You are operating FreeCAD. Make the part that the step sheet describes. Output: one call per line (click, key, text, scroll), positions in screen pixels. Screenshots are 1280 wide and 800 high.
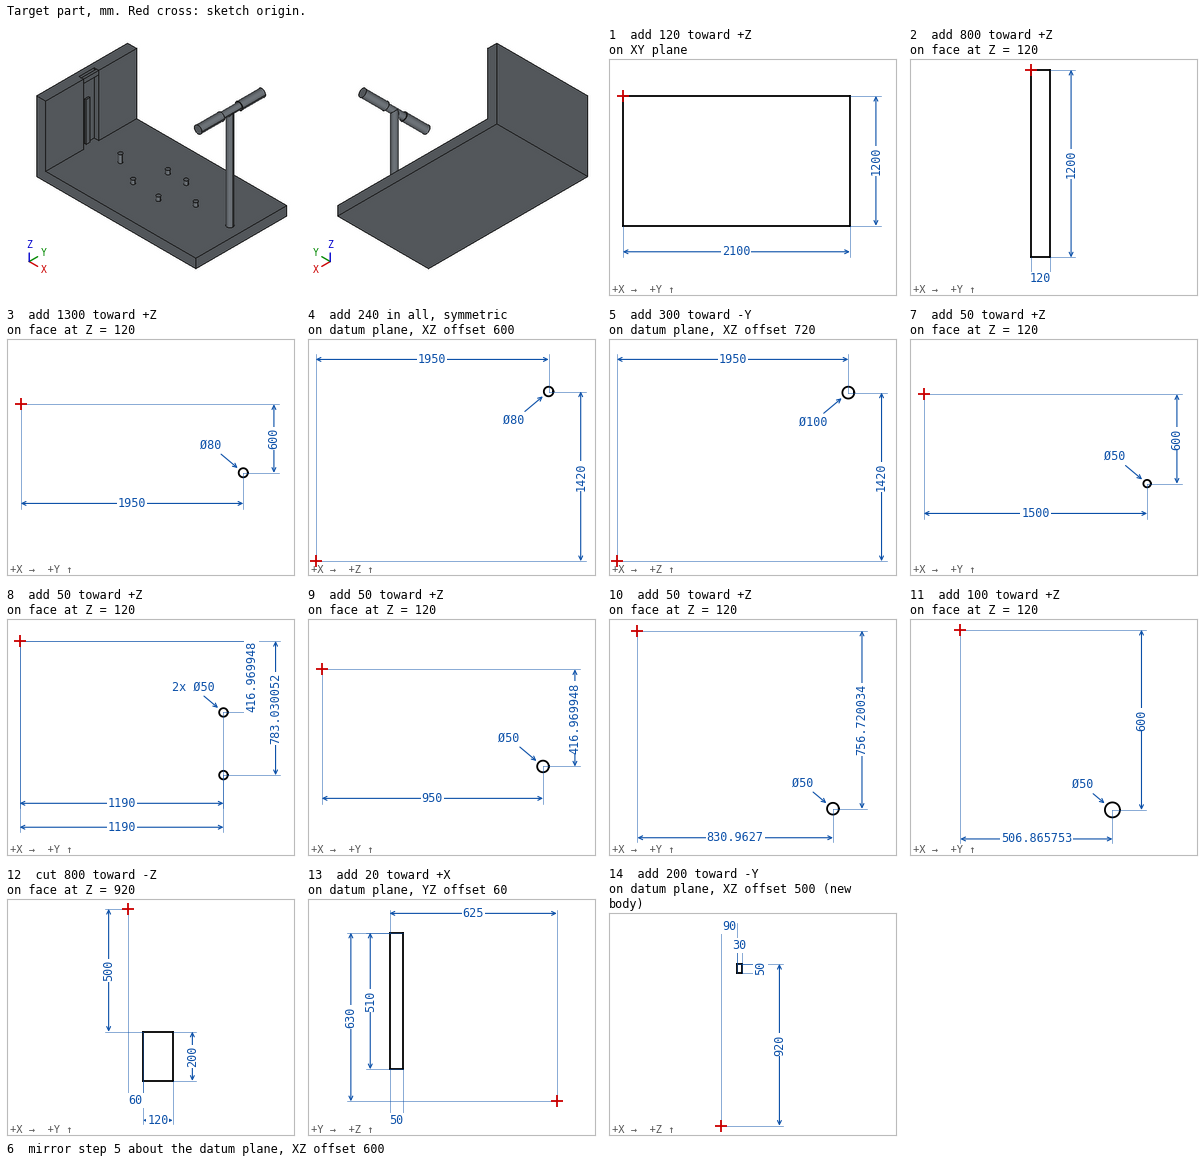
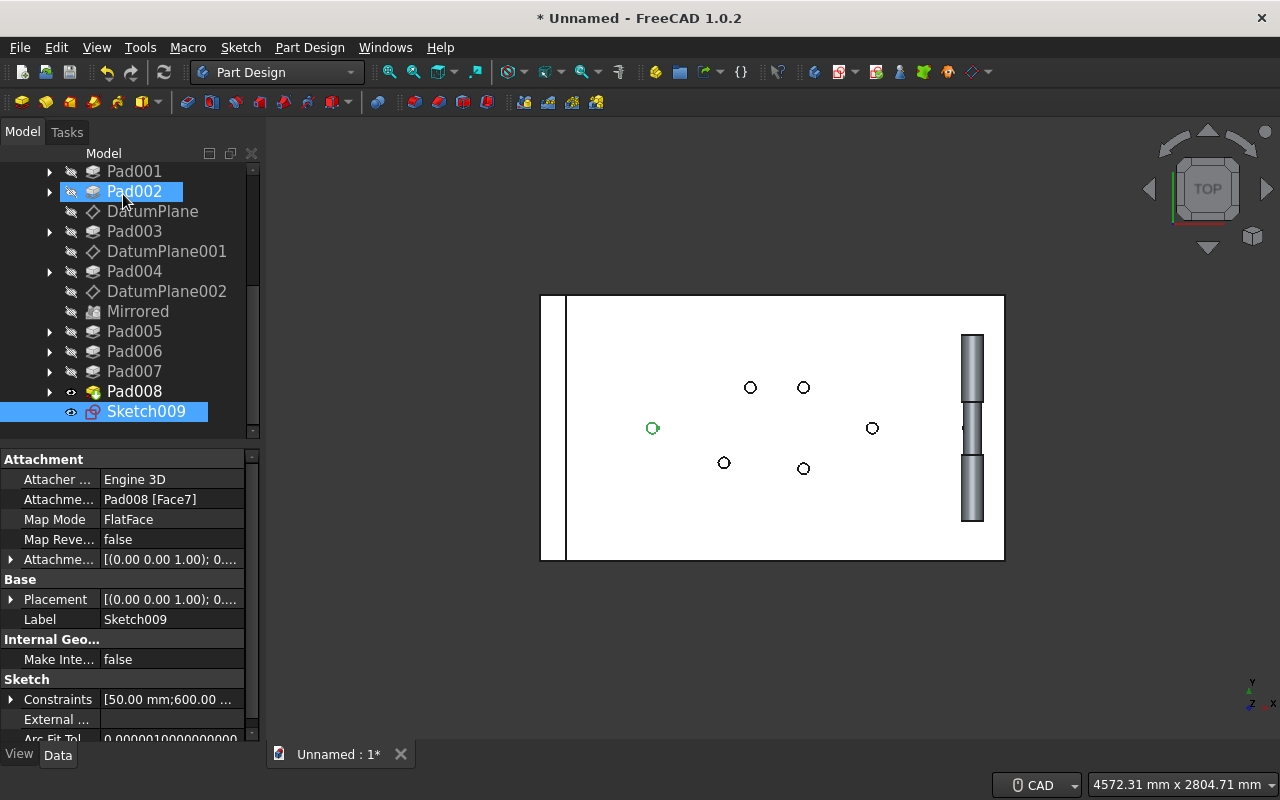
click(22, 102)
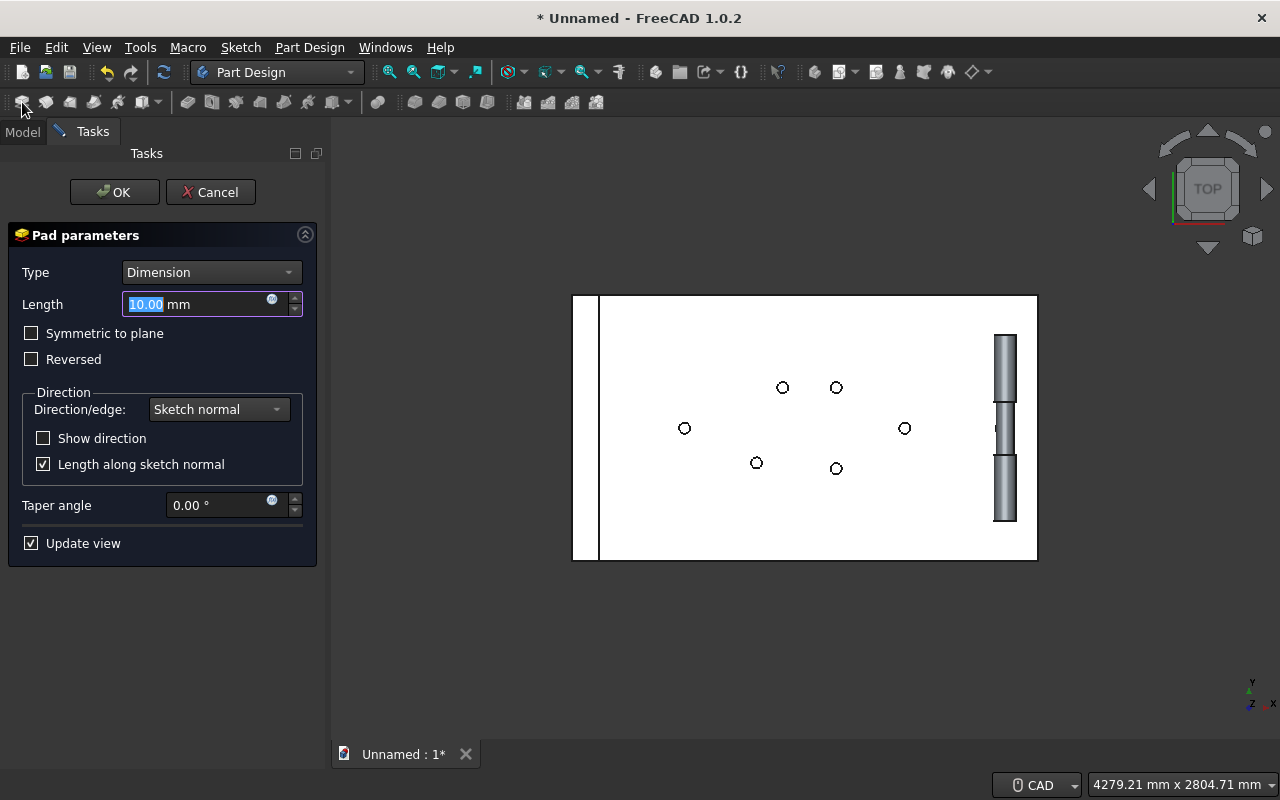
text(100)
key(Tab)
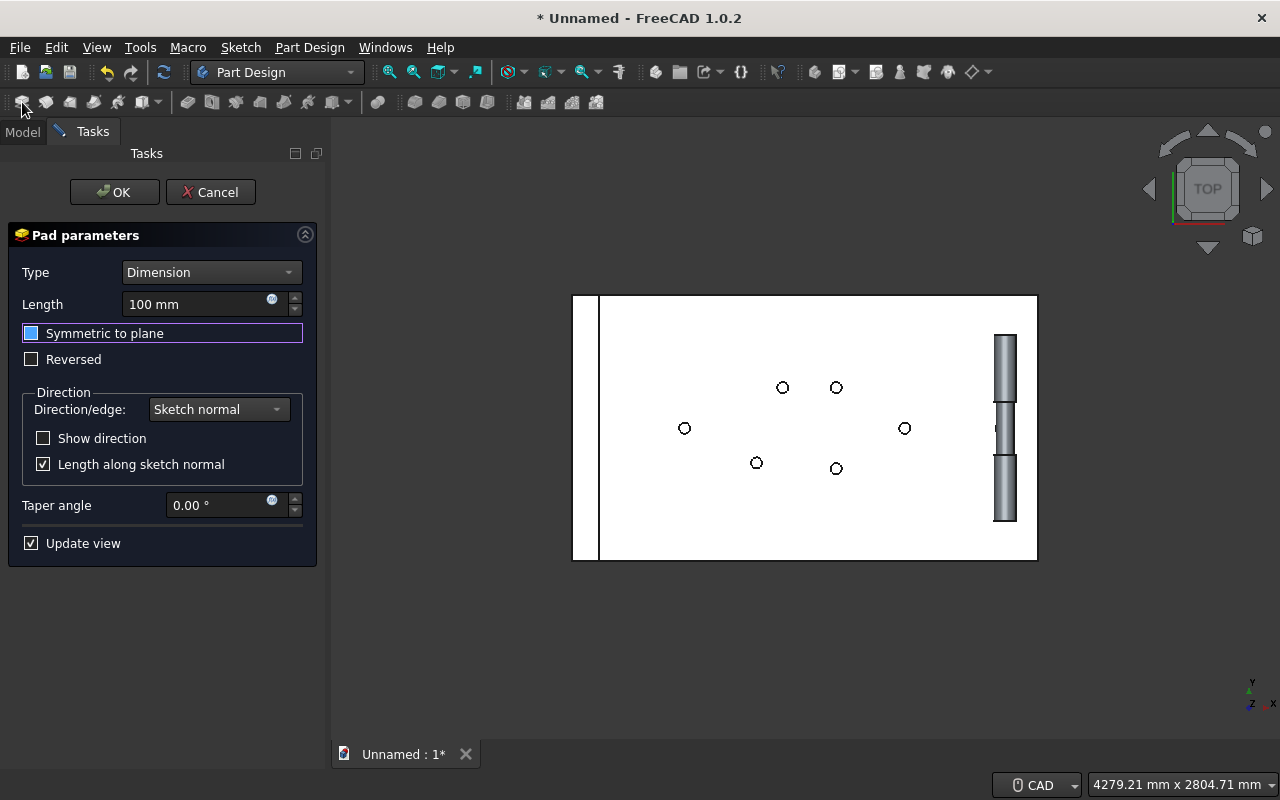
click(115, 192)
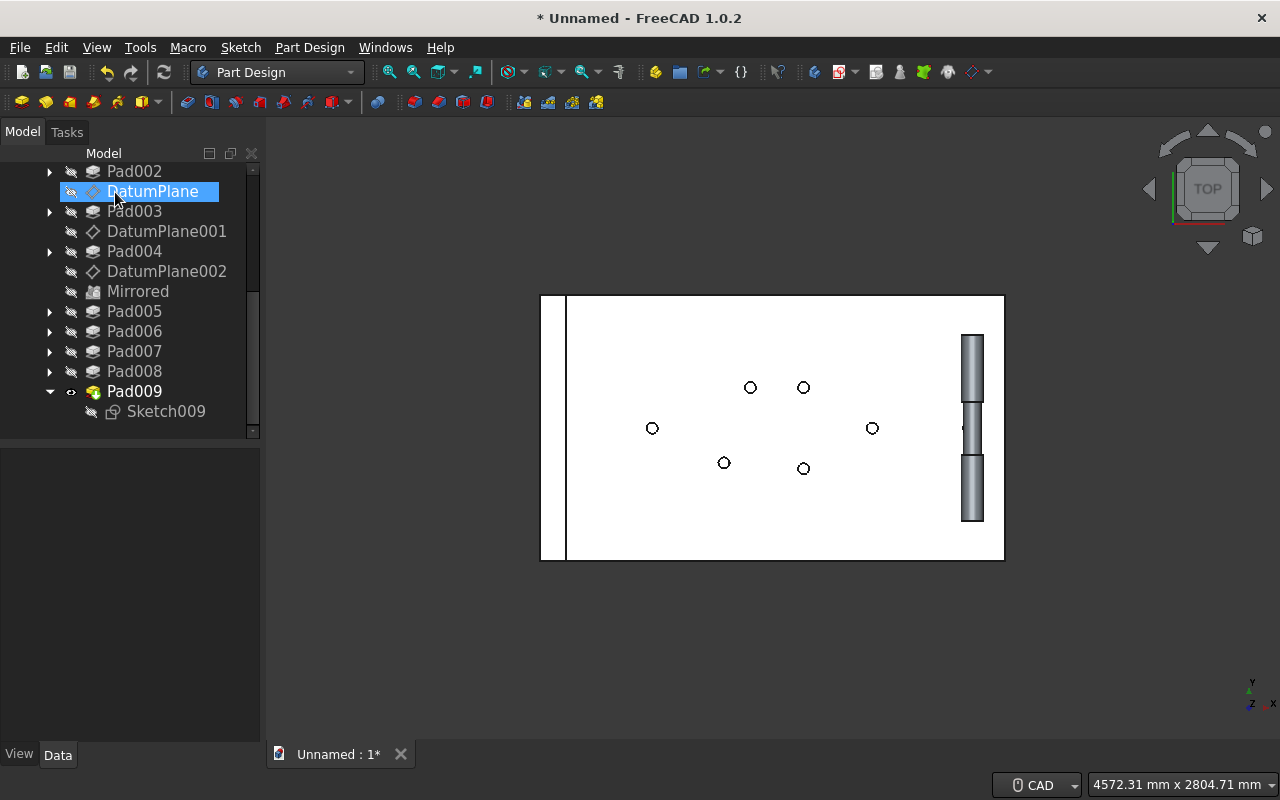
click(553, 313)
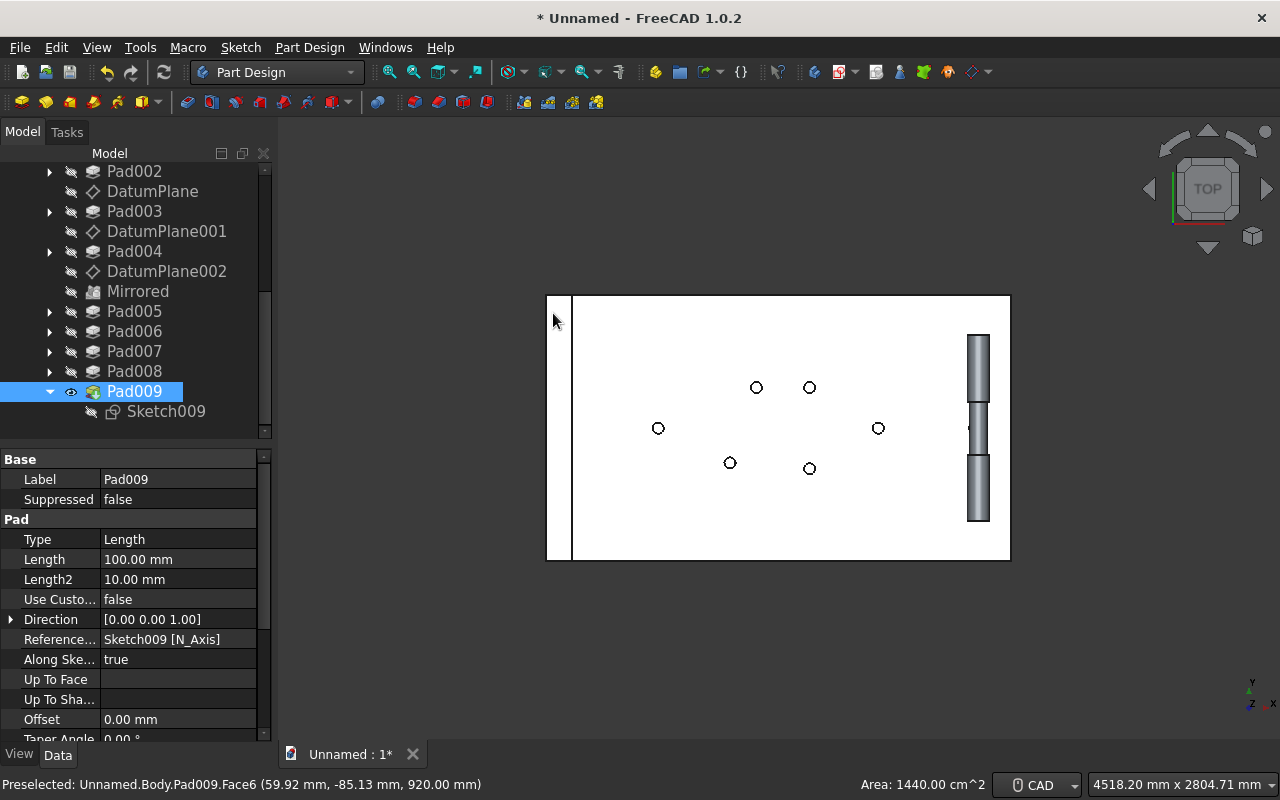
click(840, 72)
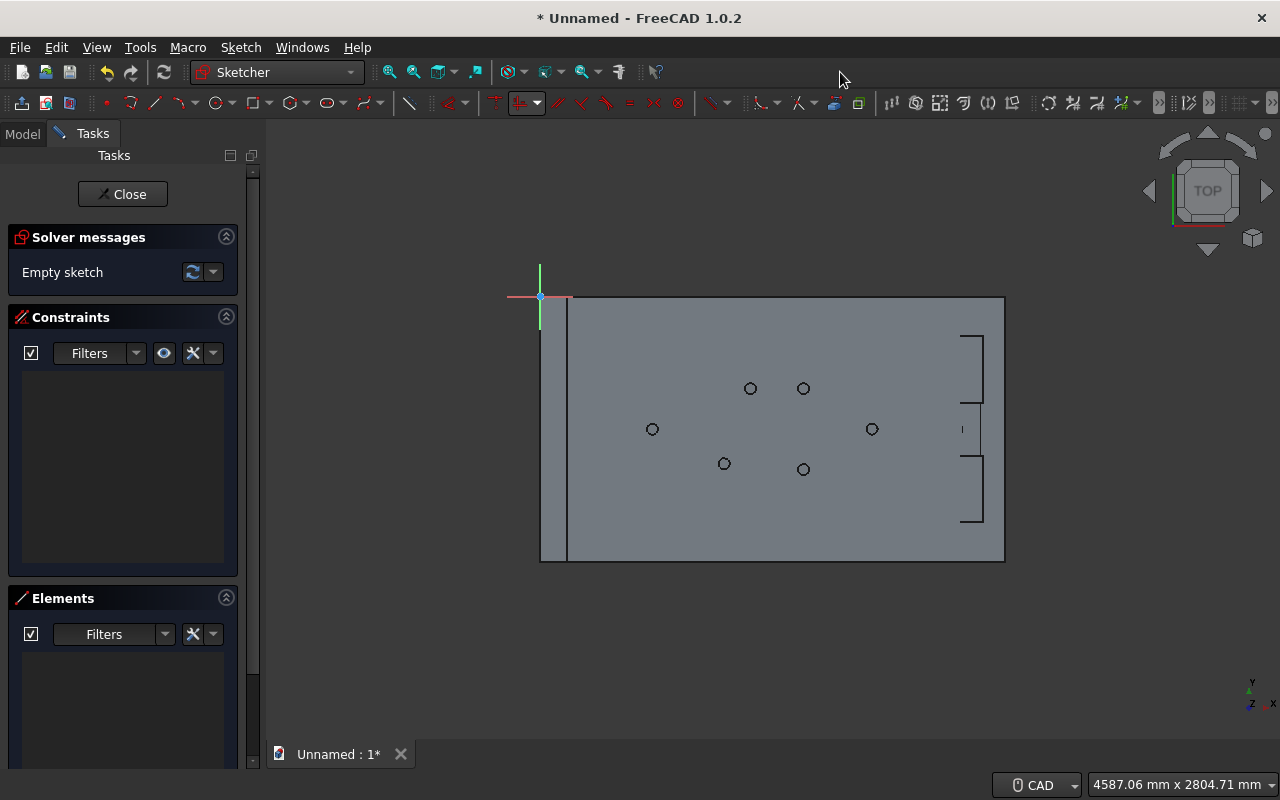
scroll(550, 429, up, 11)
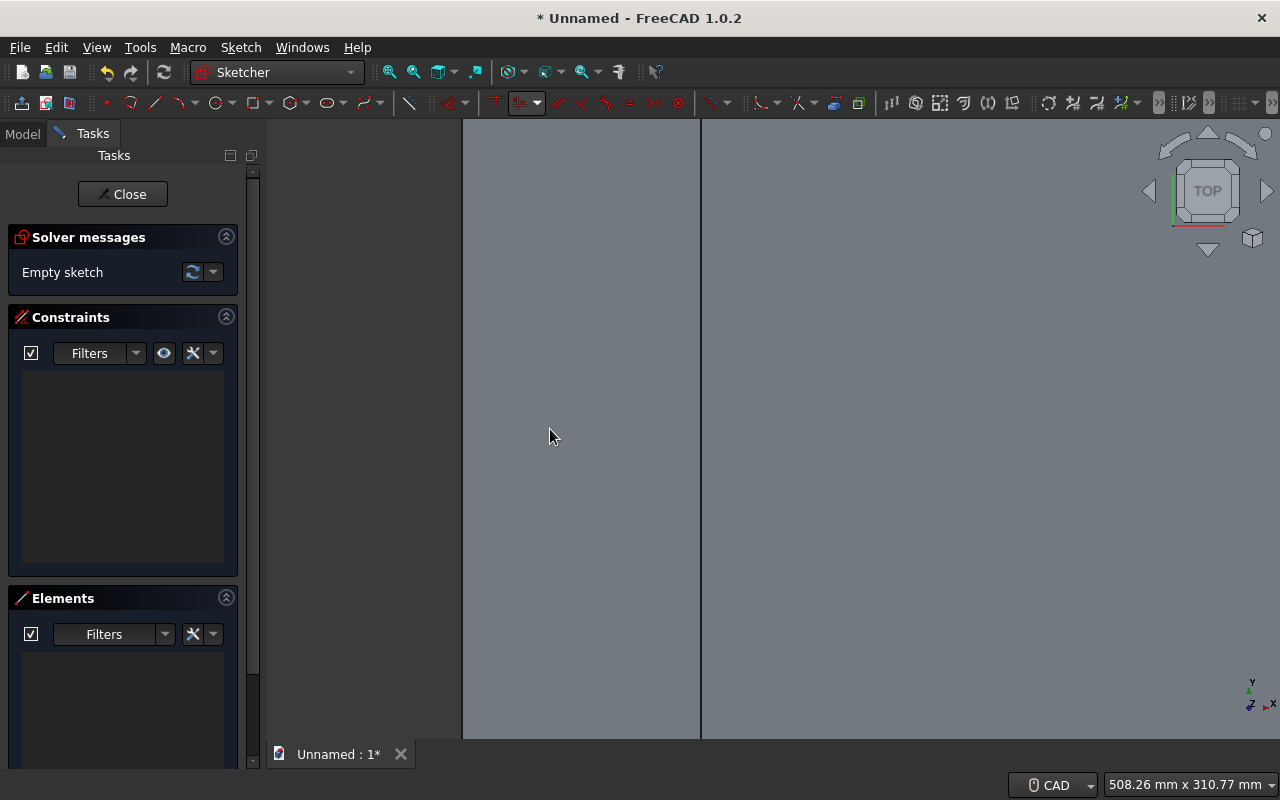
click(254, 104)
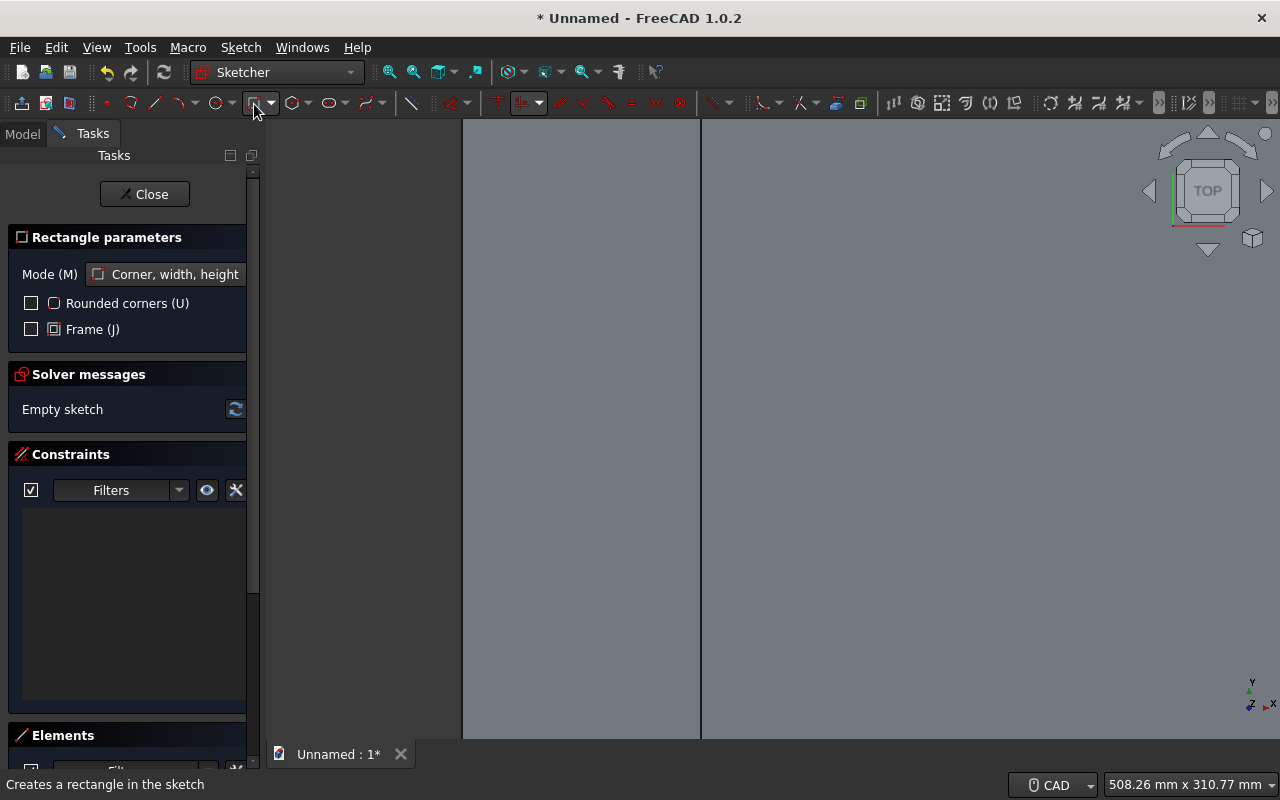
click(581, 227)
move(821, 626)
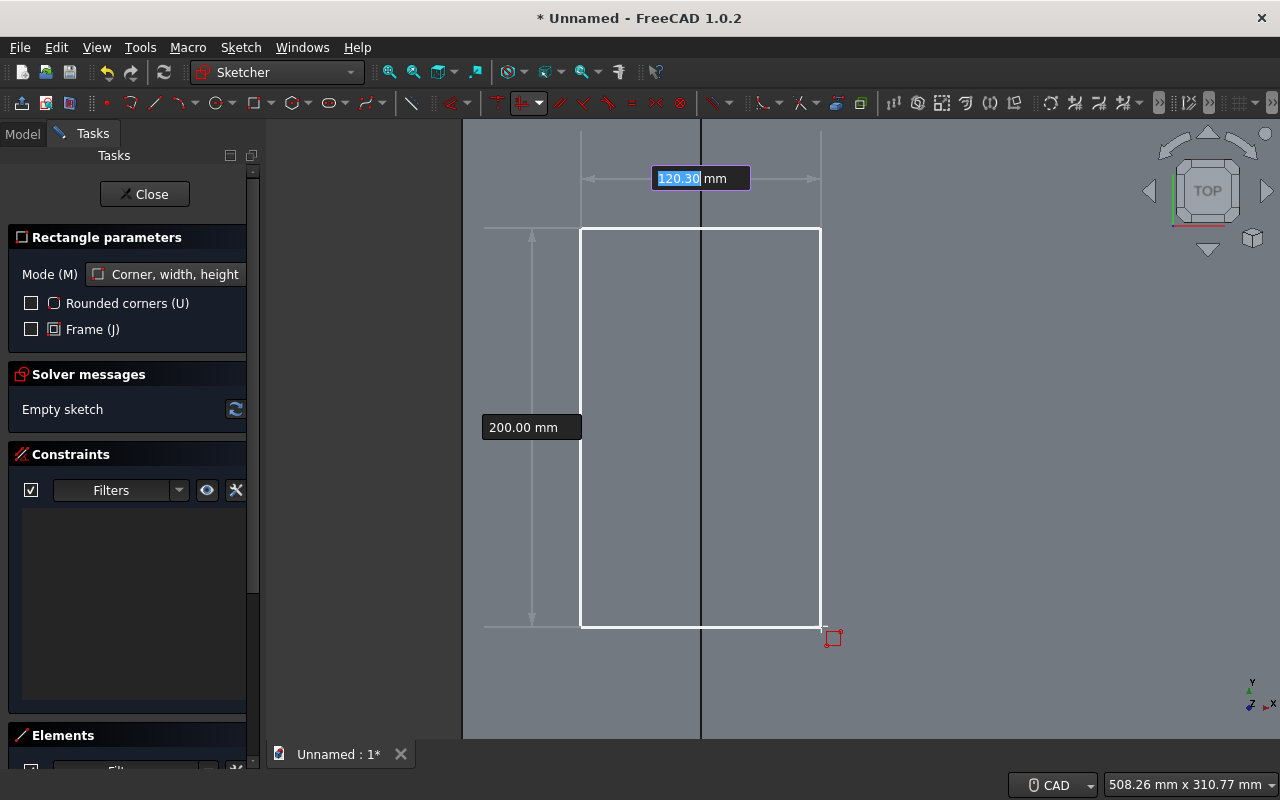
text(120)
key(Tab)
text(200)
key(Return)
key(Escape)